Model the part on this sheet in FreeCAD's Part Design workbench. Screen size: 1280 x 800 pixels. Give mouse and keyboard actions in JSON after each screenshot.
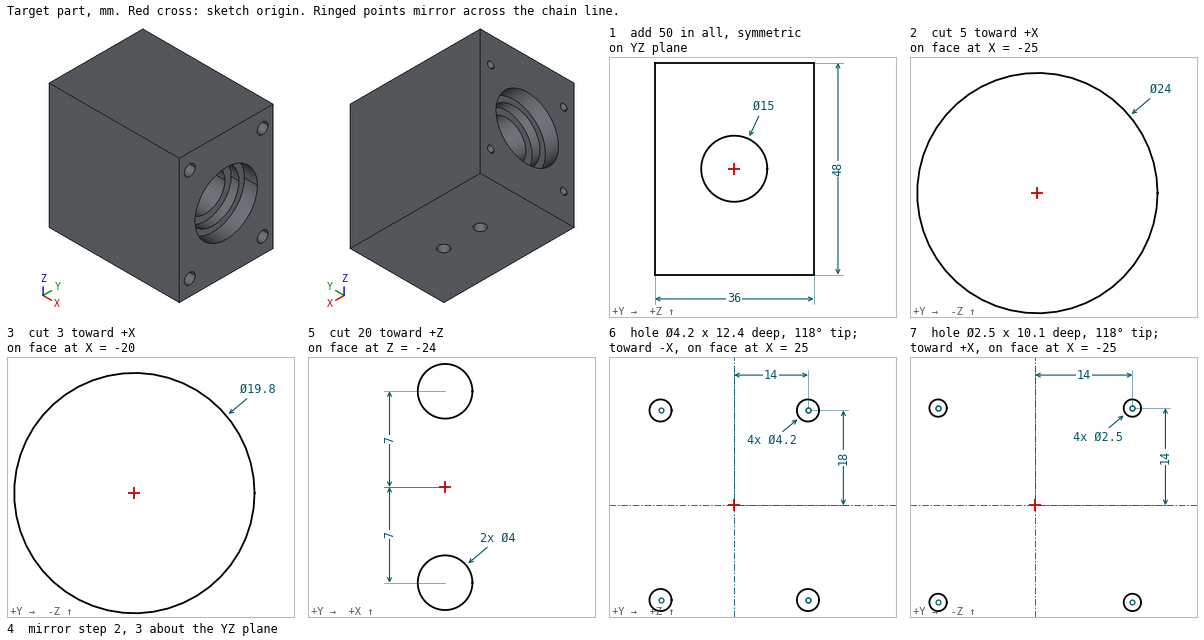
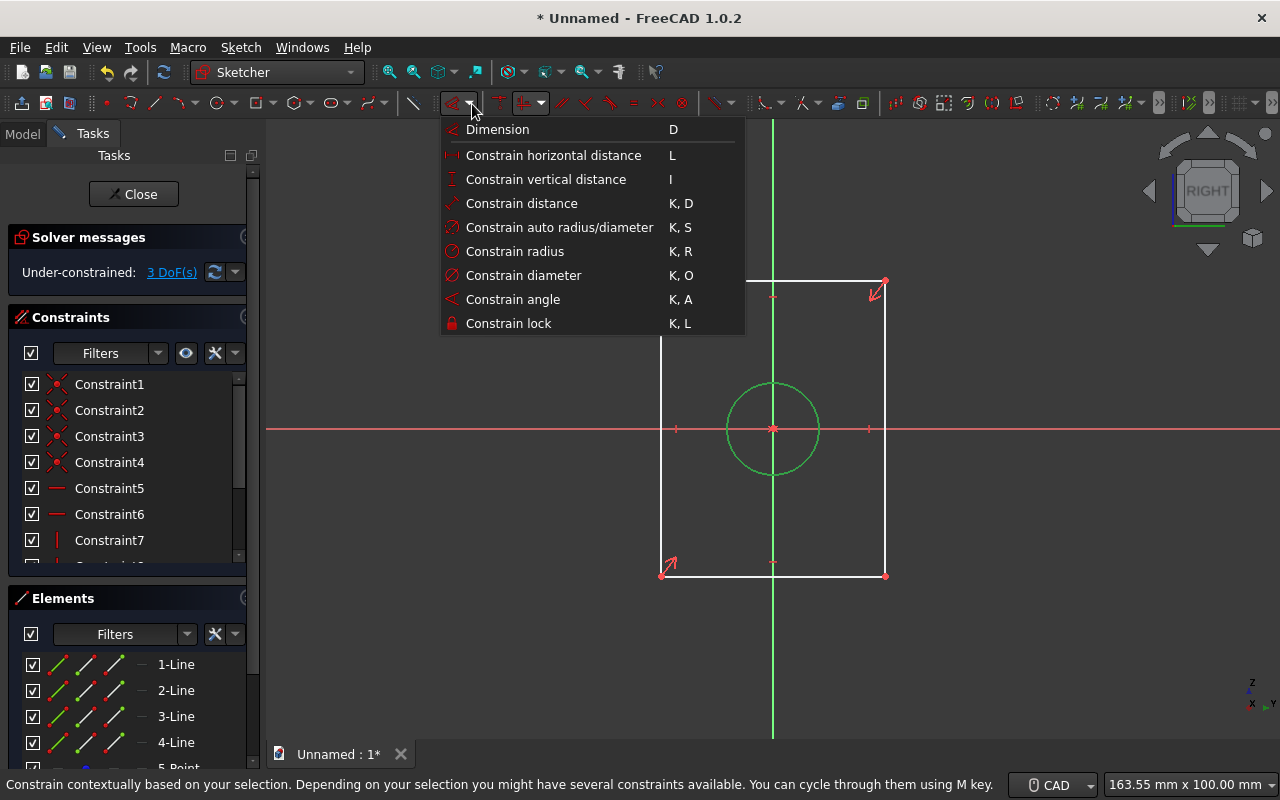
{"action": "left_click", "coordinate": [593, 275]}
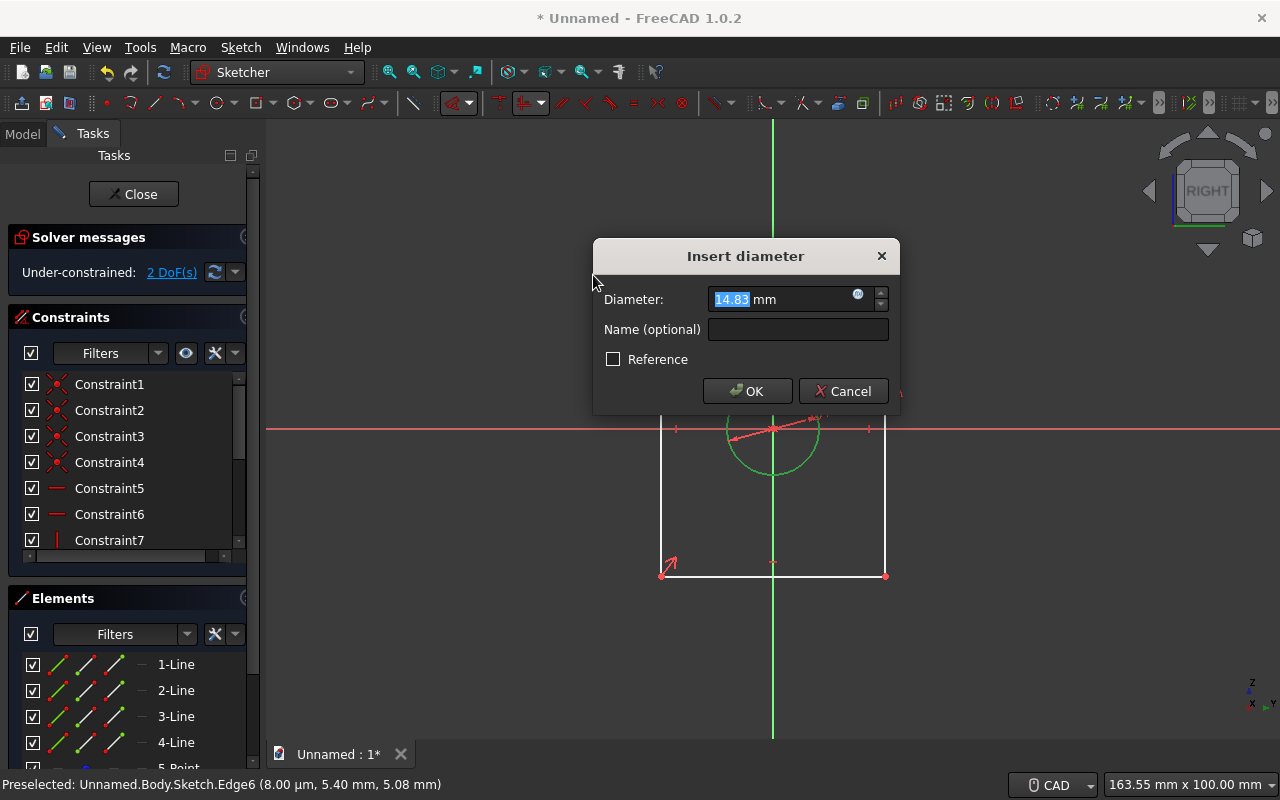
{"action": "type", "text": "15"}
{"action": "key", "text": "Return"}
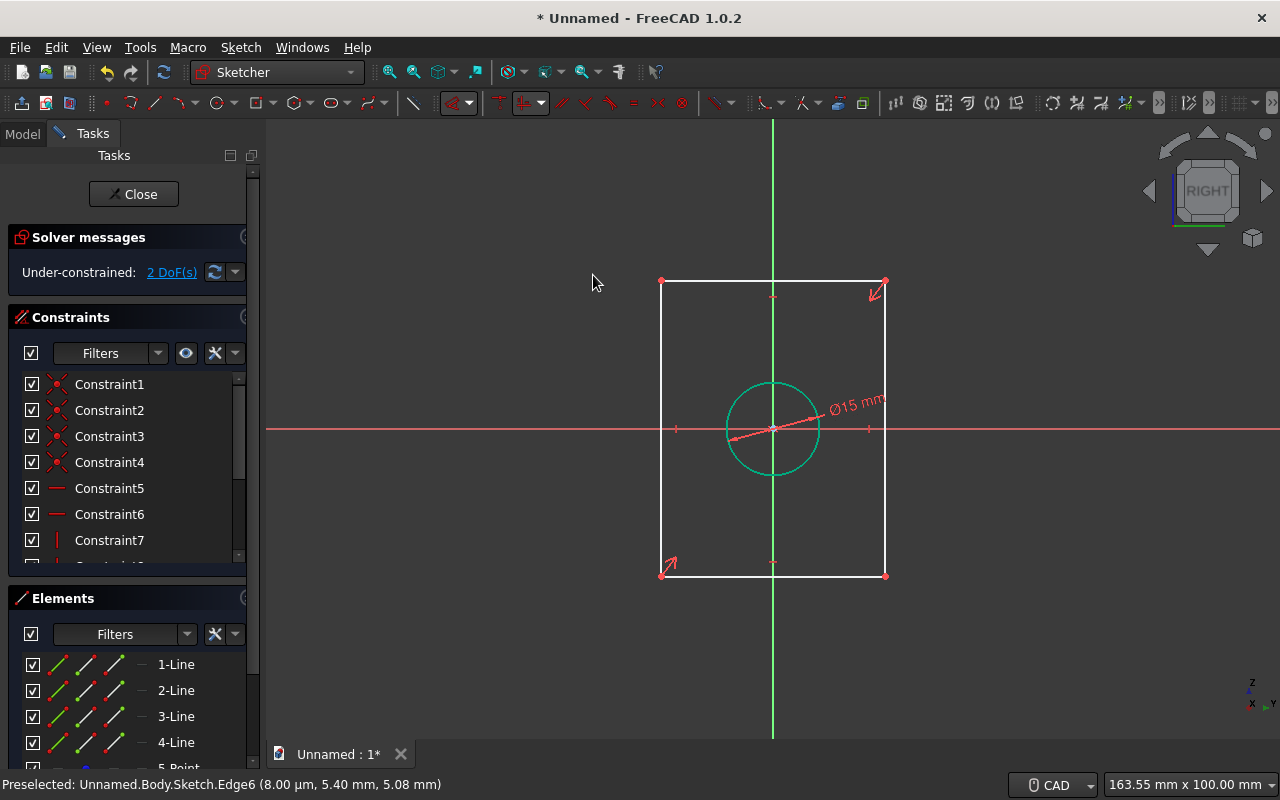
{"action": "left_click", "coordinate": [728, 577]}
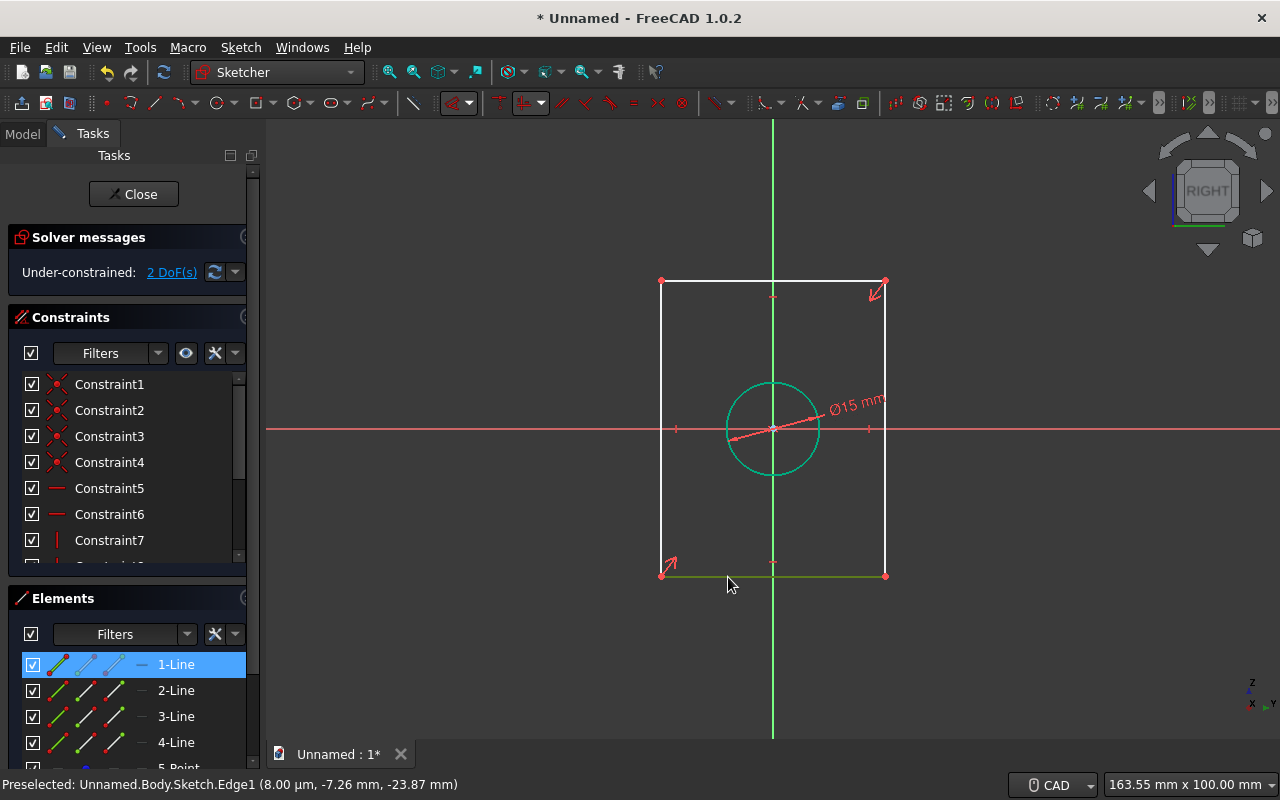
{"action": "left_click", "coordinate": [472, 104]}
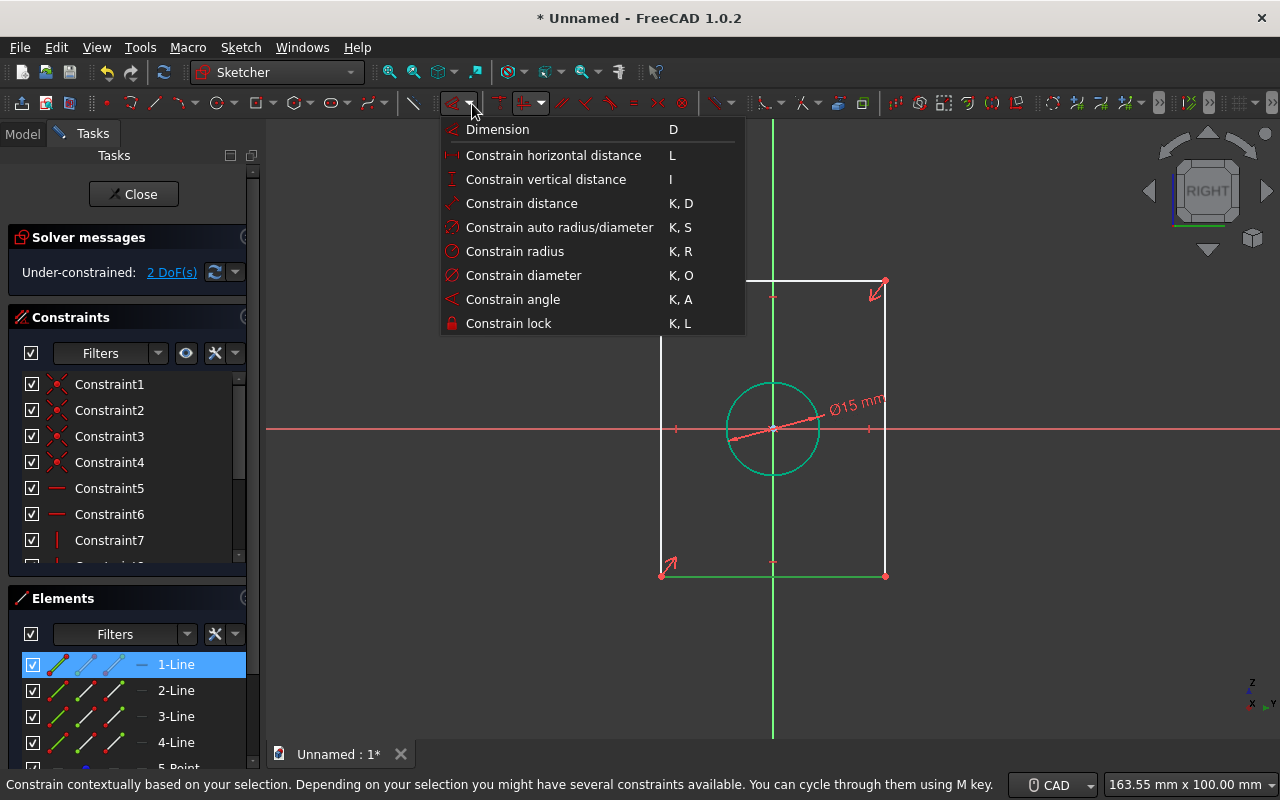
{"action": "left_click", "coordinate": [593, 155]}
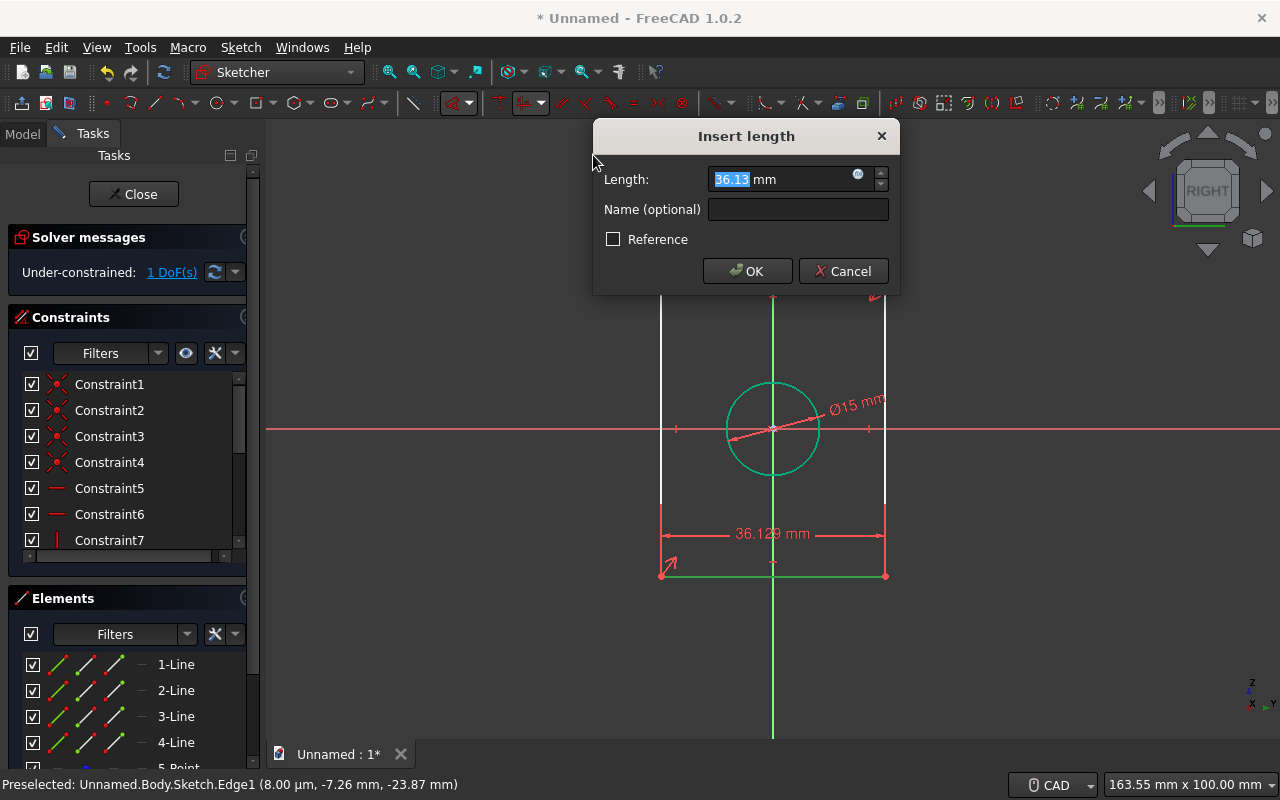
{"action": "type", "text": "36"}
{"action": "key", "text": "Return"}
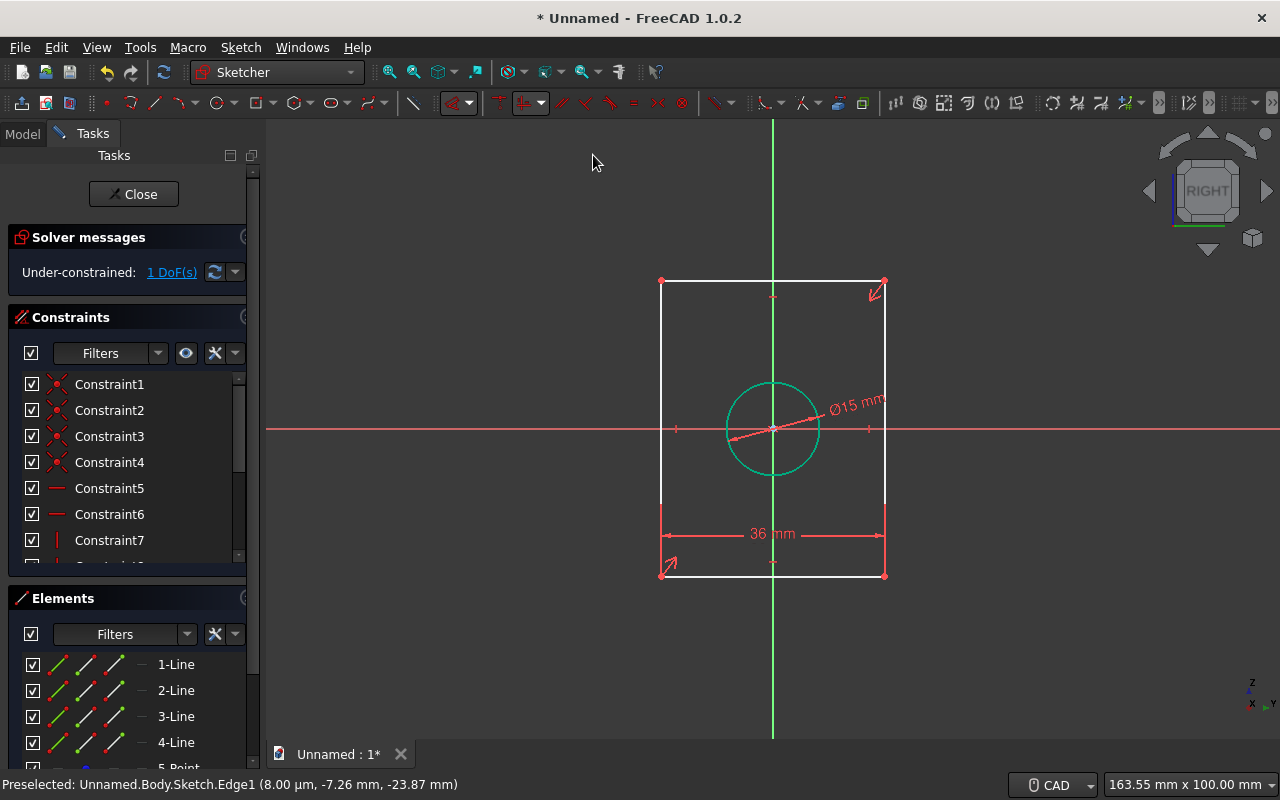
{"action": "left_click", "coordinate": [885, 488]}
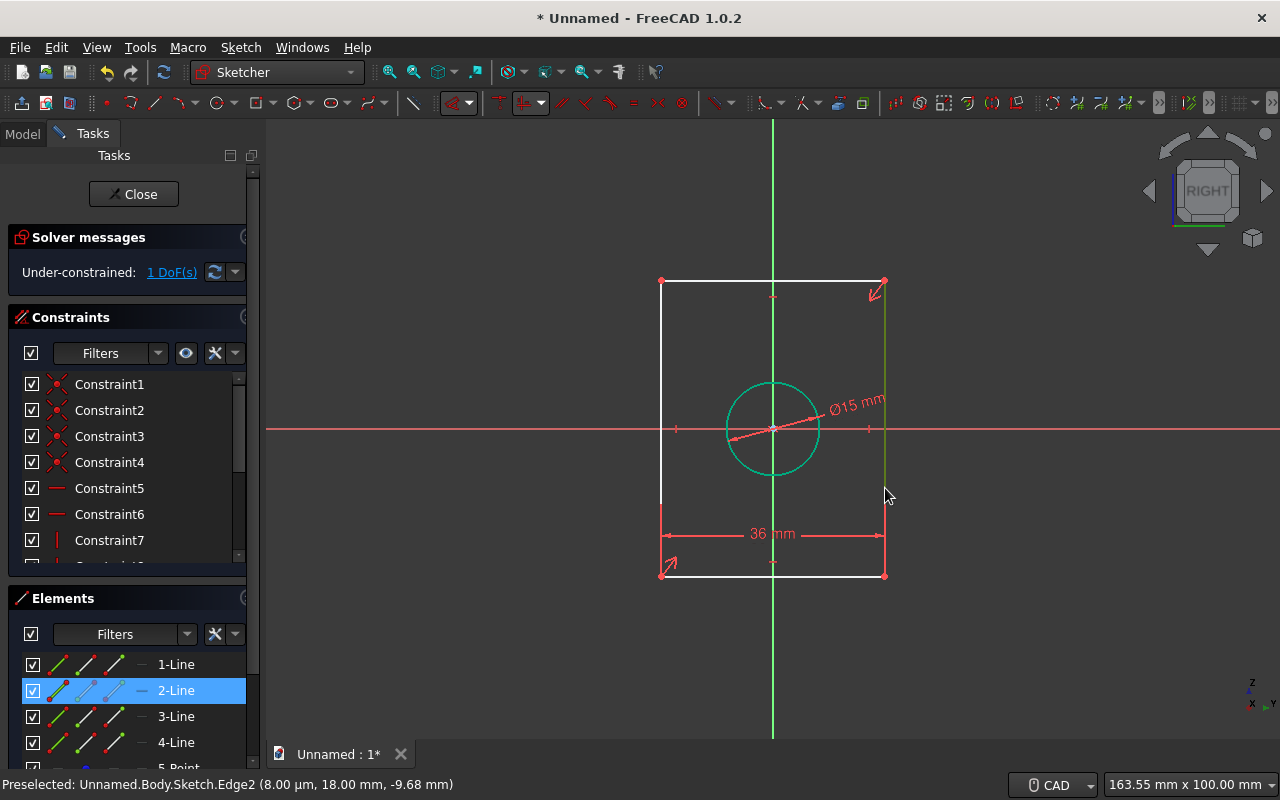
{"action": "left_click", "coordinate": [472, 104]}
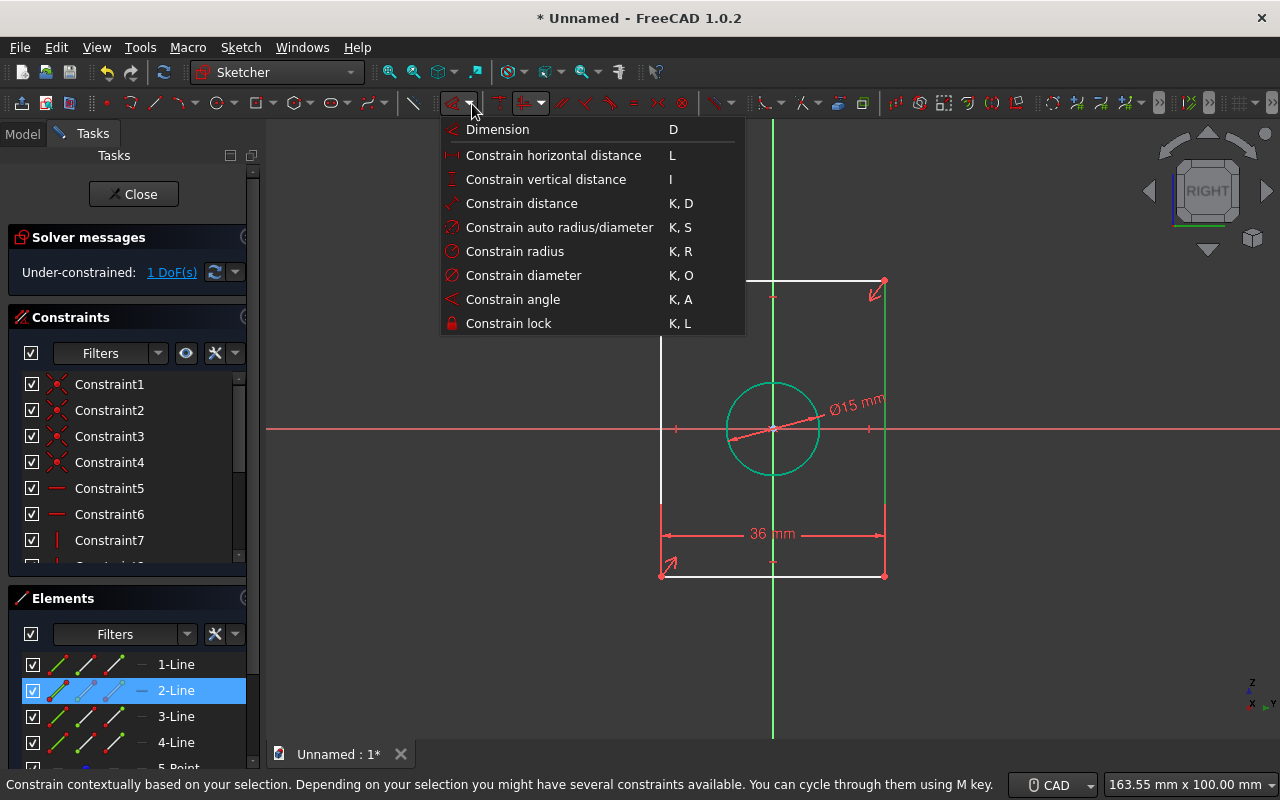
{"action": "left_click", "coordinate": [593, 179]}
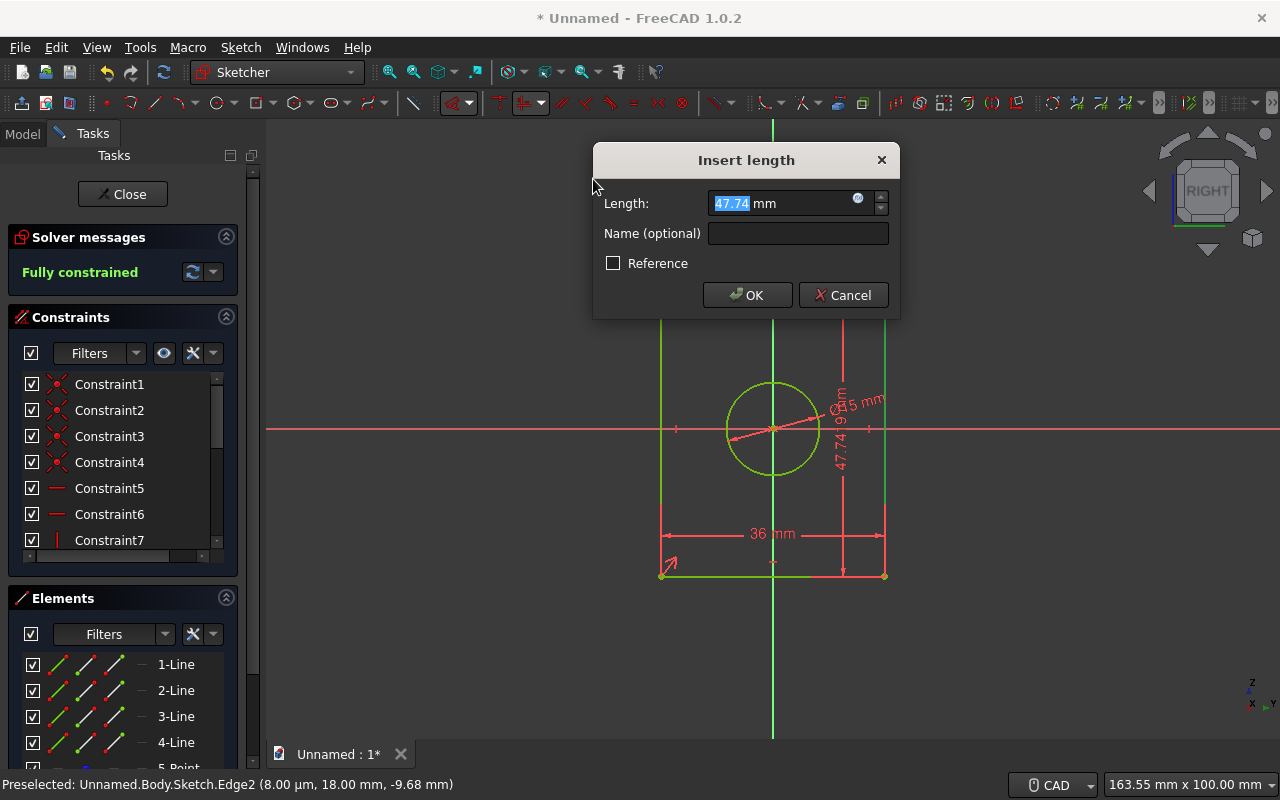
{"action": "type", "text": "48"}
{"action": "key", "text": "Return"}